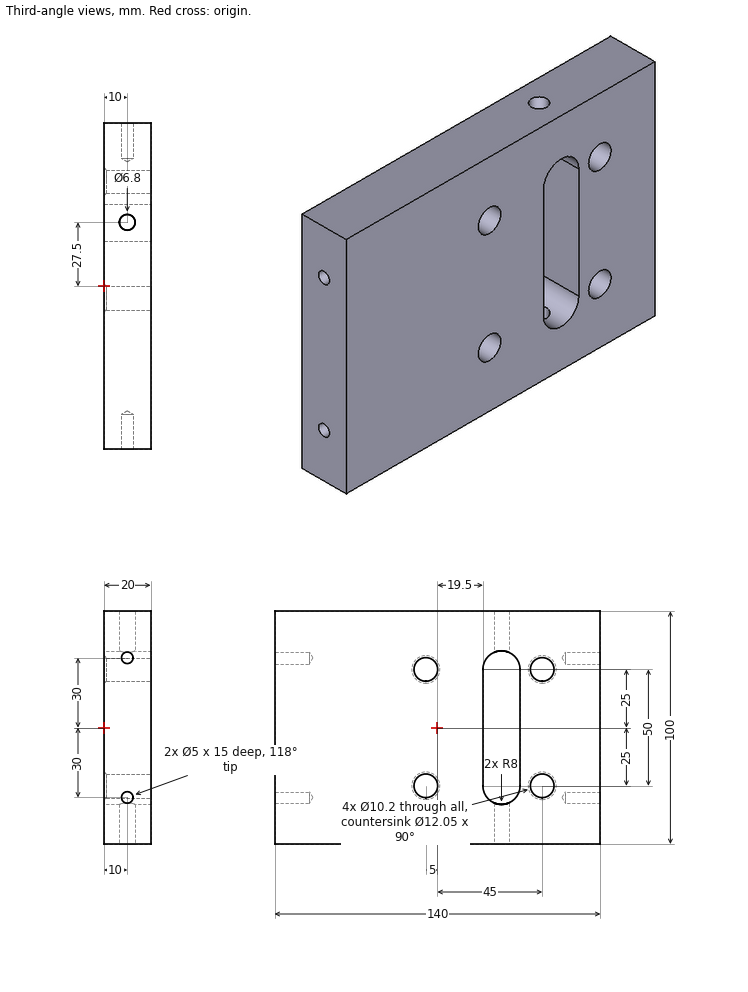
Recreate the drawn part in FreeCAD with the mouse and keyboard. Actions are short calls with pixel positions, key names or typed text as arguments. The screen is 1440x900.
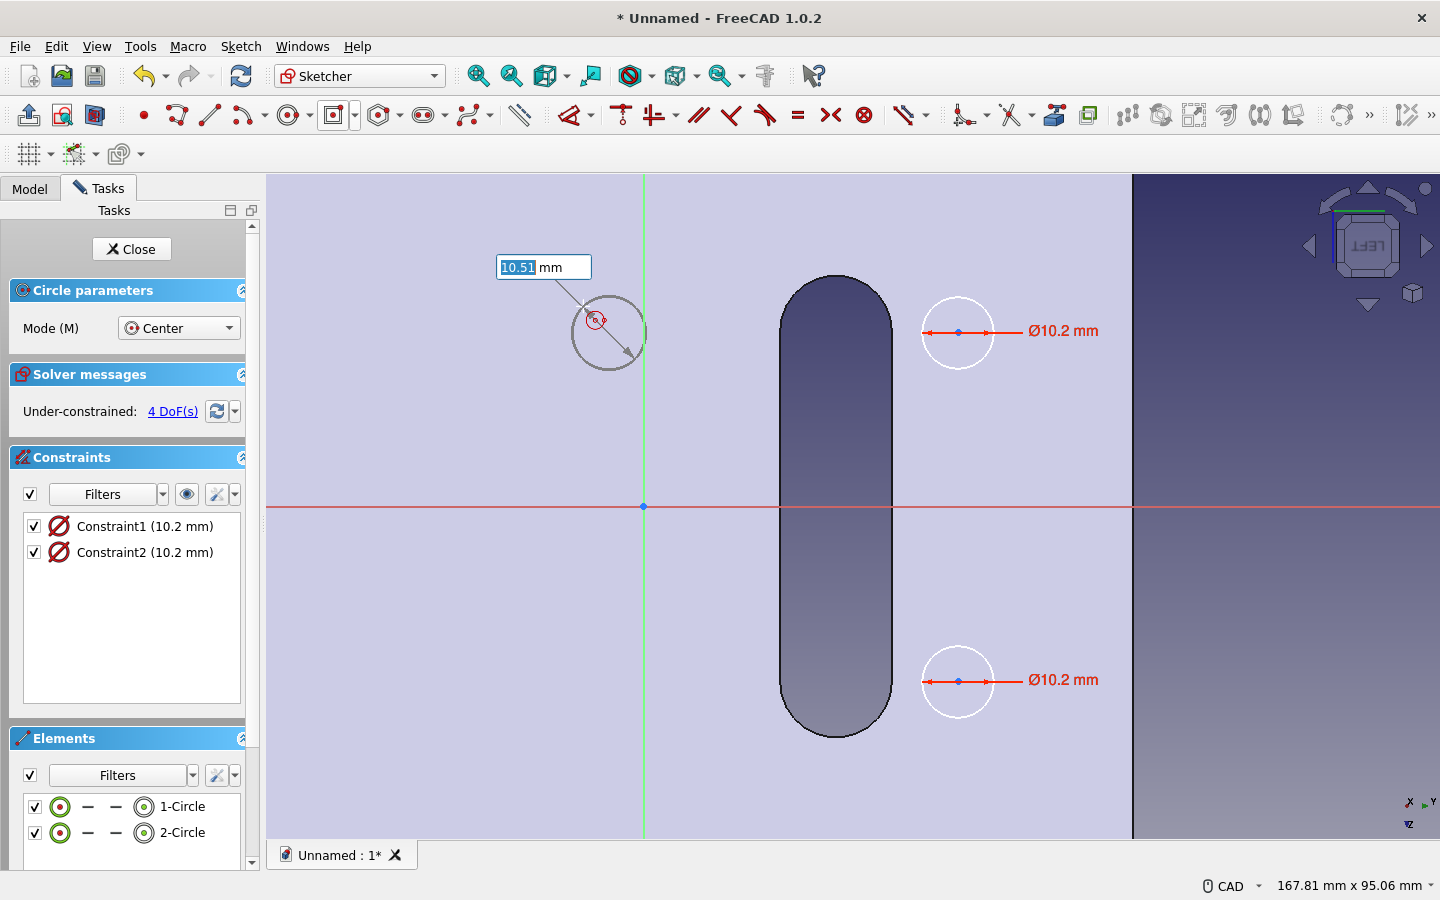
text(10.2)
key(Return)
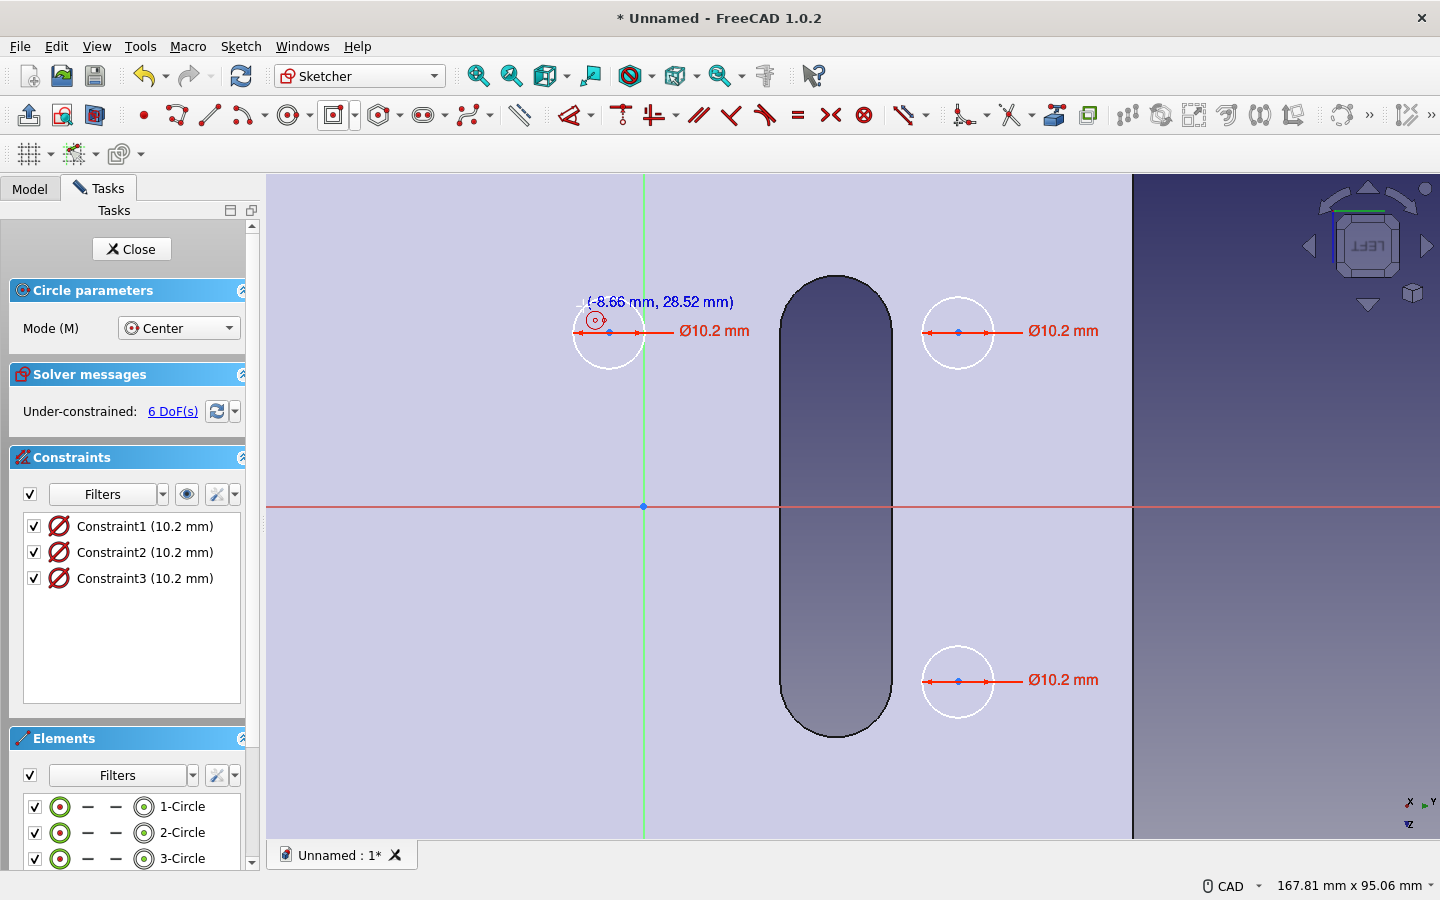
click(609, 681)
move(583, 656)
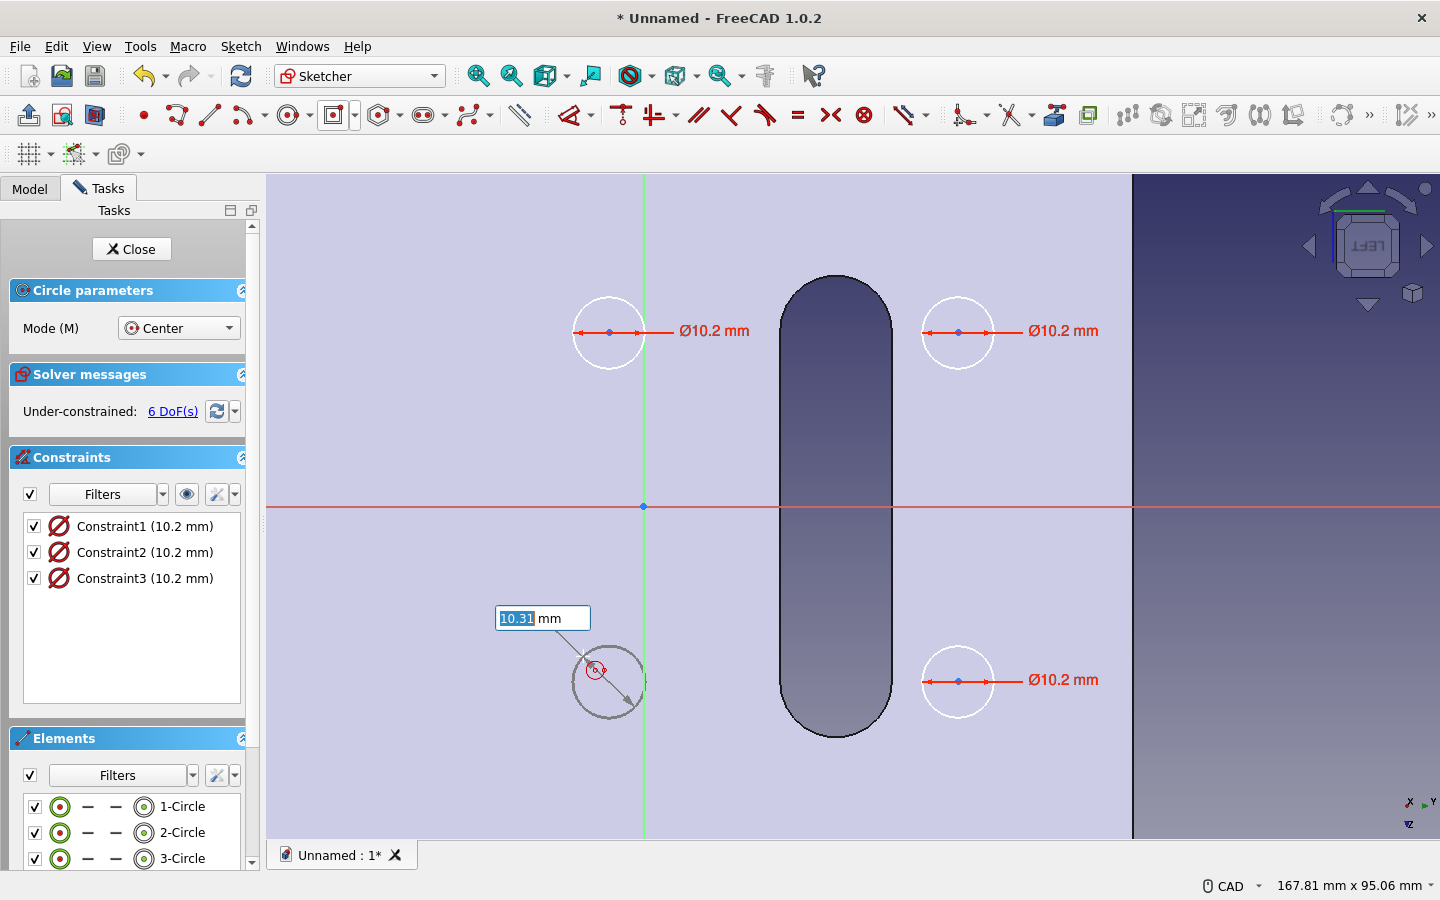
text(10.2)
key(Return)
key(Escape)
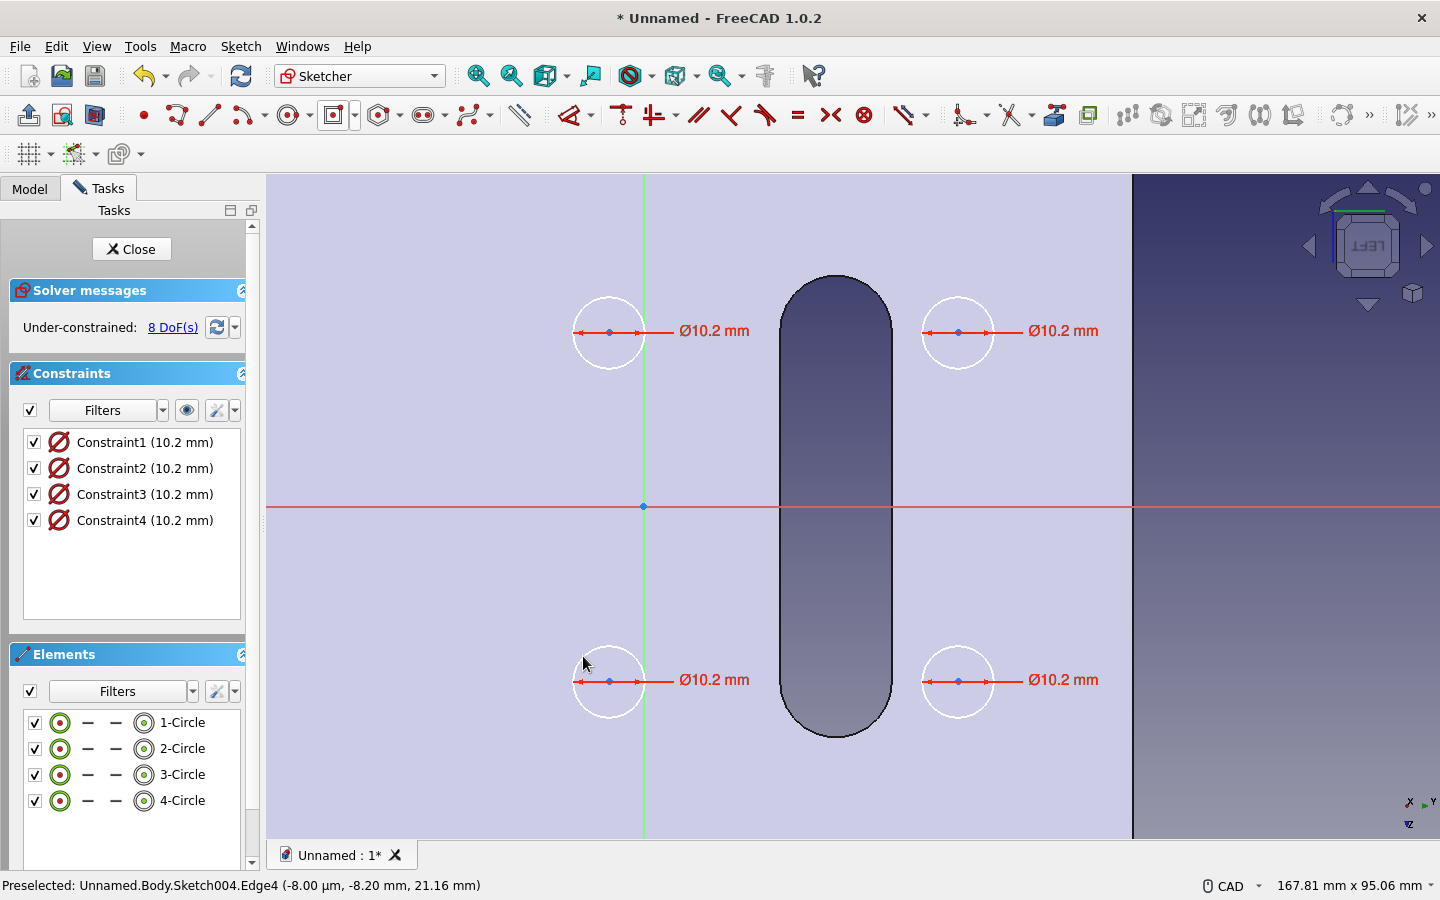
click(958, 333)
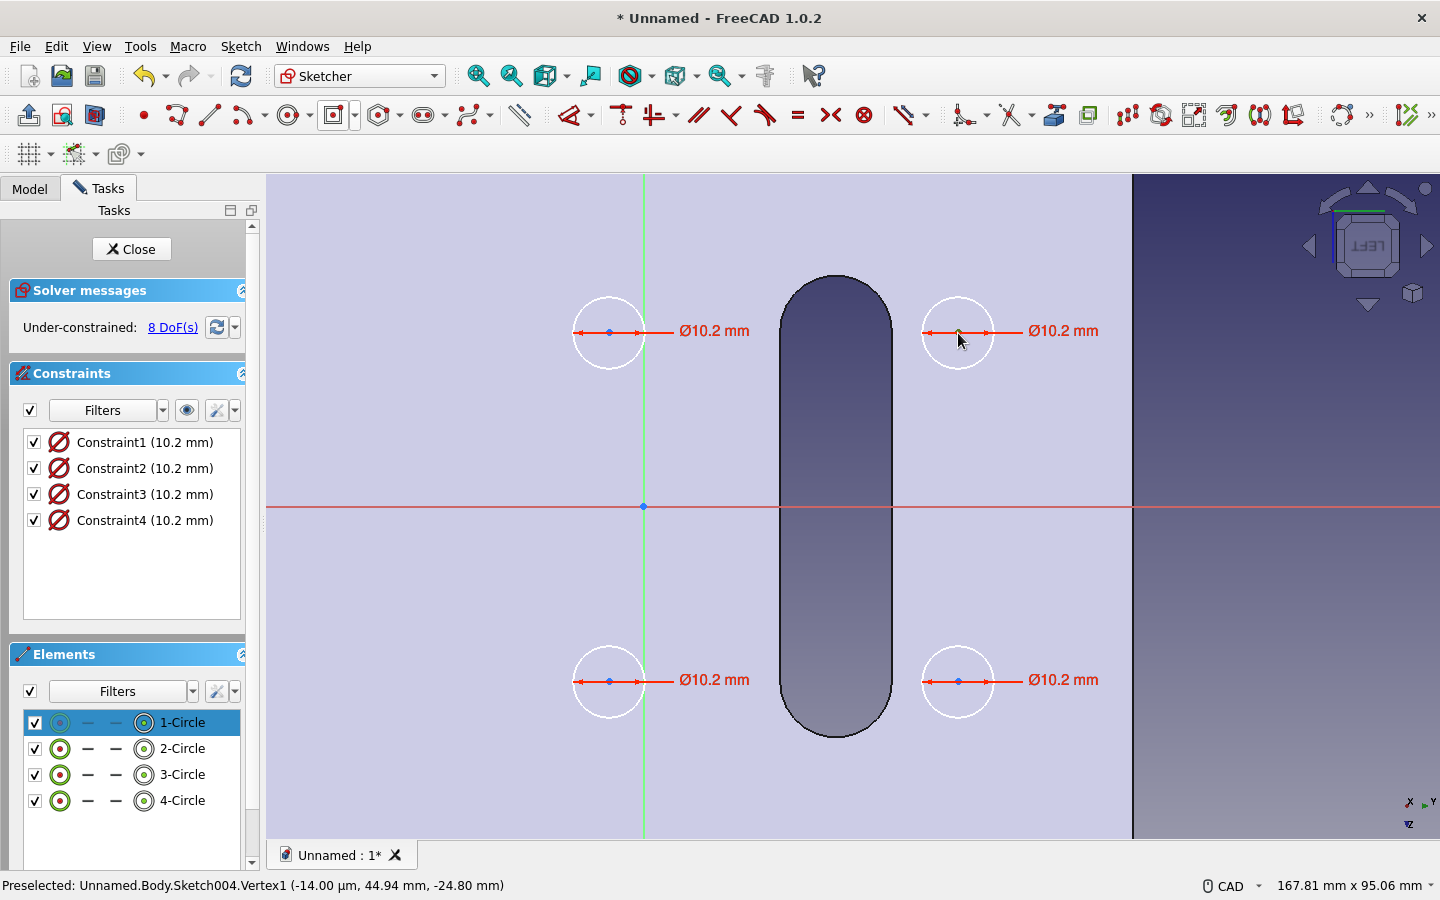
click(958, 682)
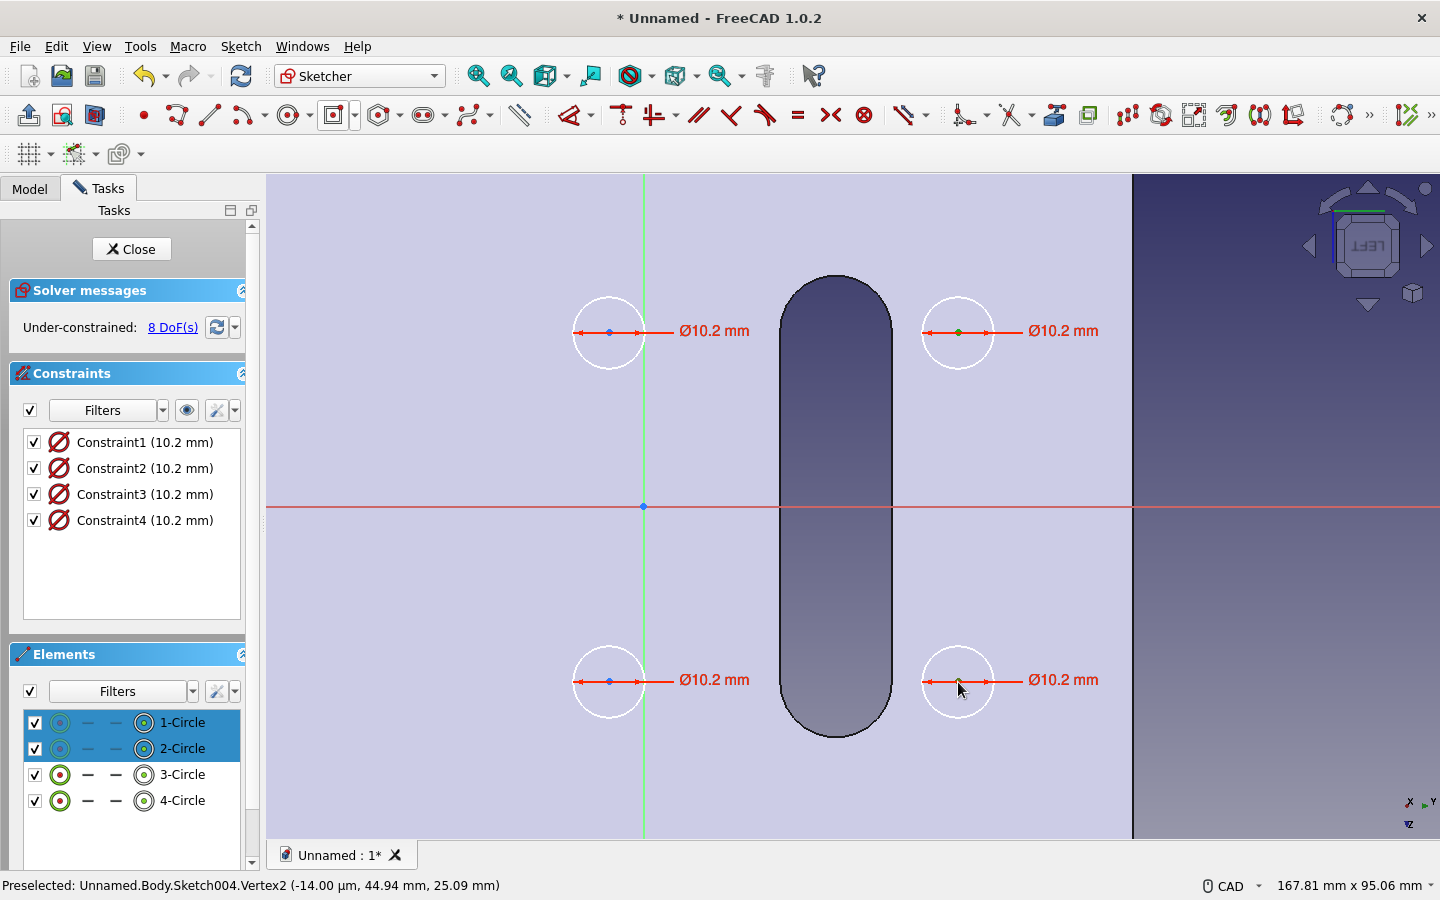
click(676, 116)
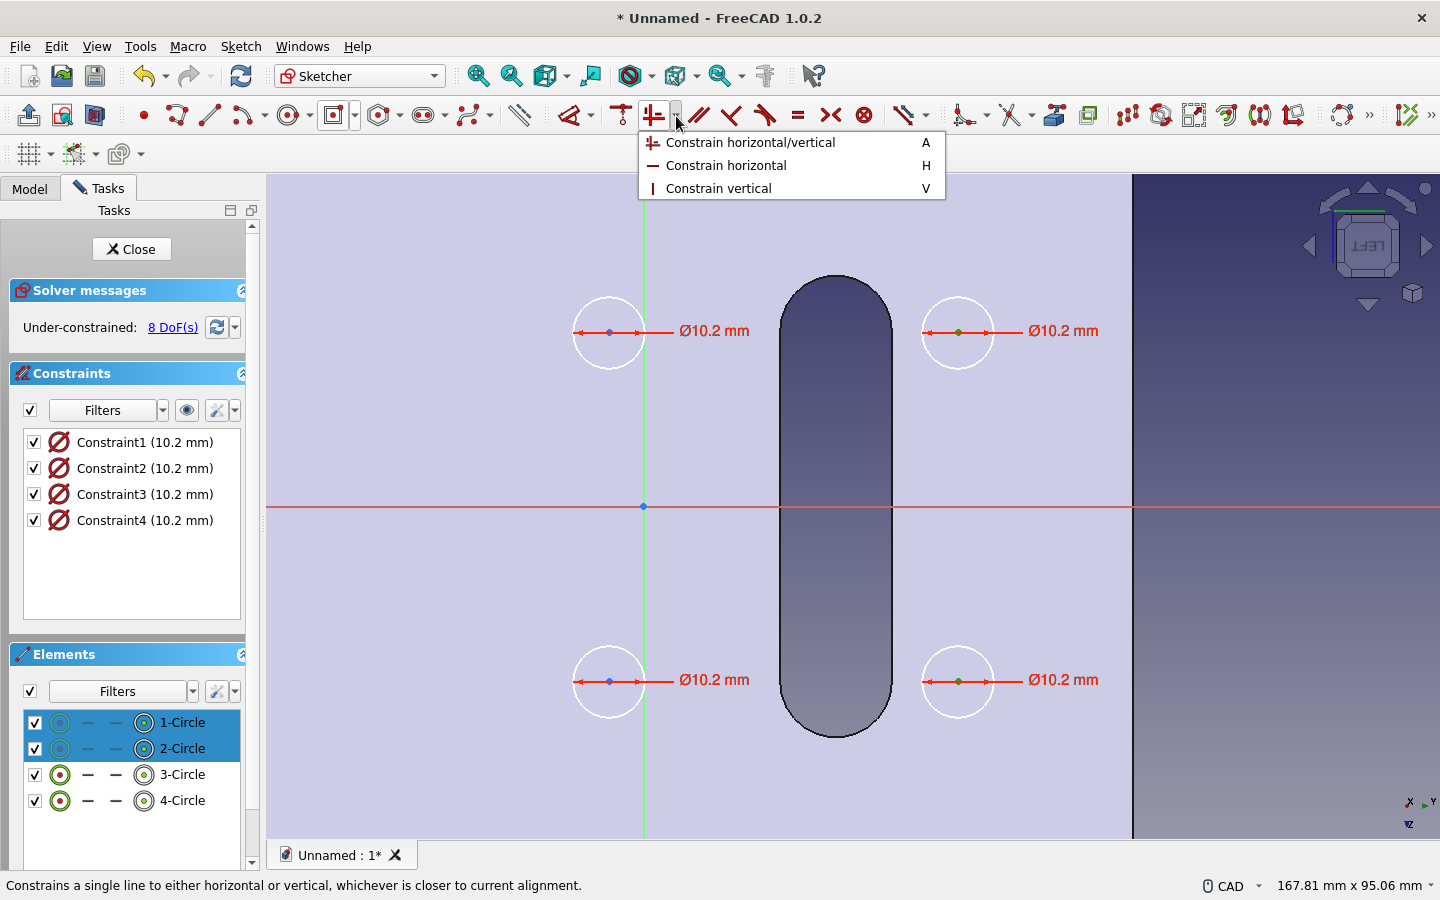
click(792, 188)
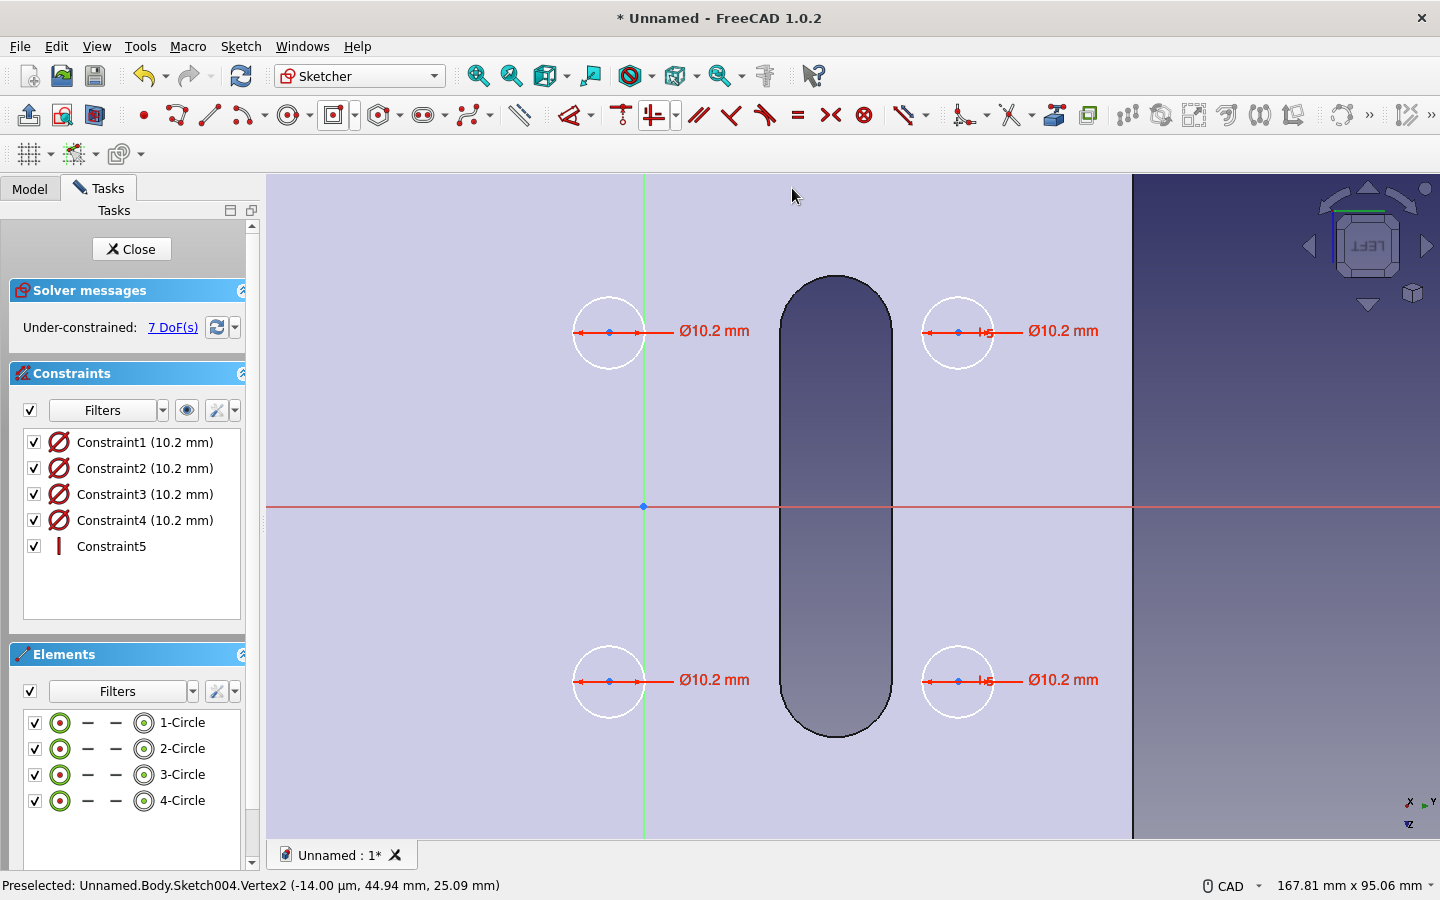
click(958, 333)